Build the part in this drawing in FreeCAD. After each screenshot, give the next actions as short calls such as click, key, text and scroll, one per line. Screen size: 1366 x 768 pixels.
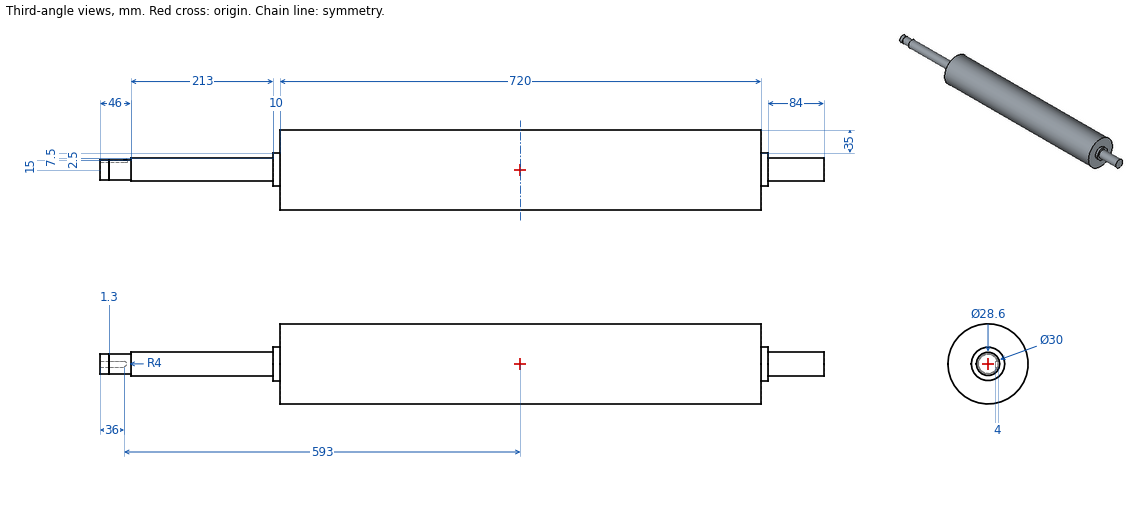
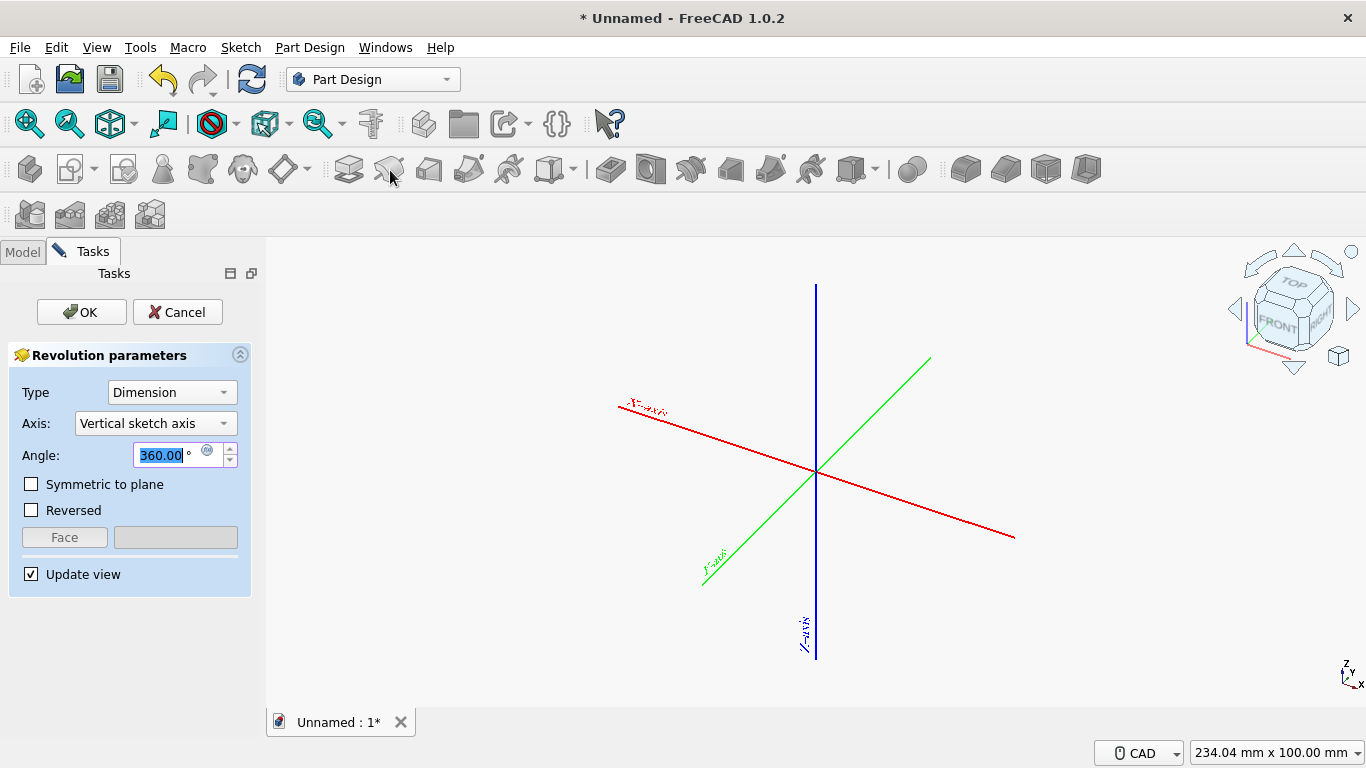
click(156, 424)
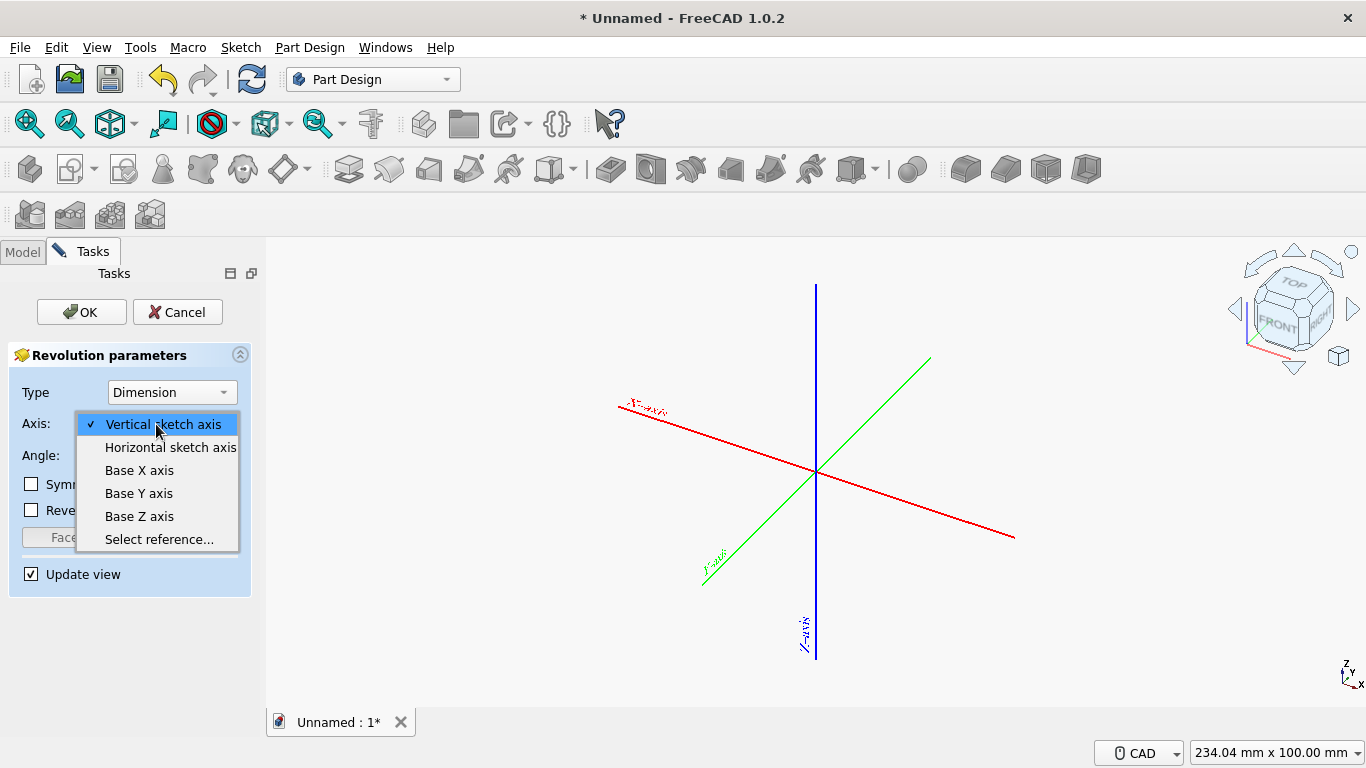
click(156, 448)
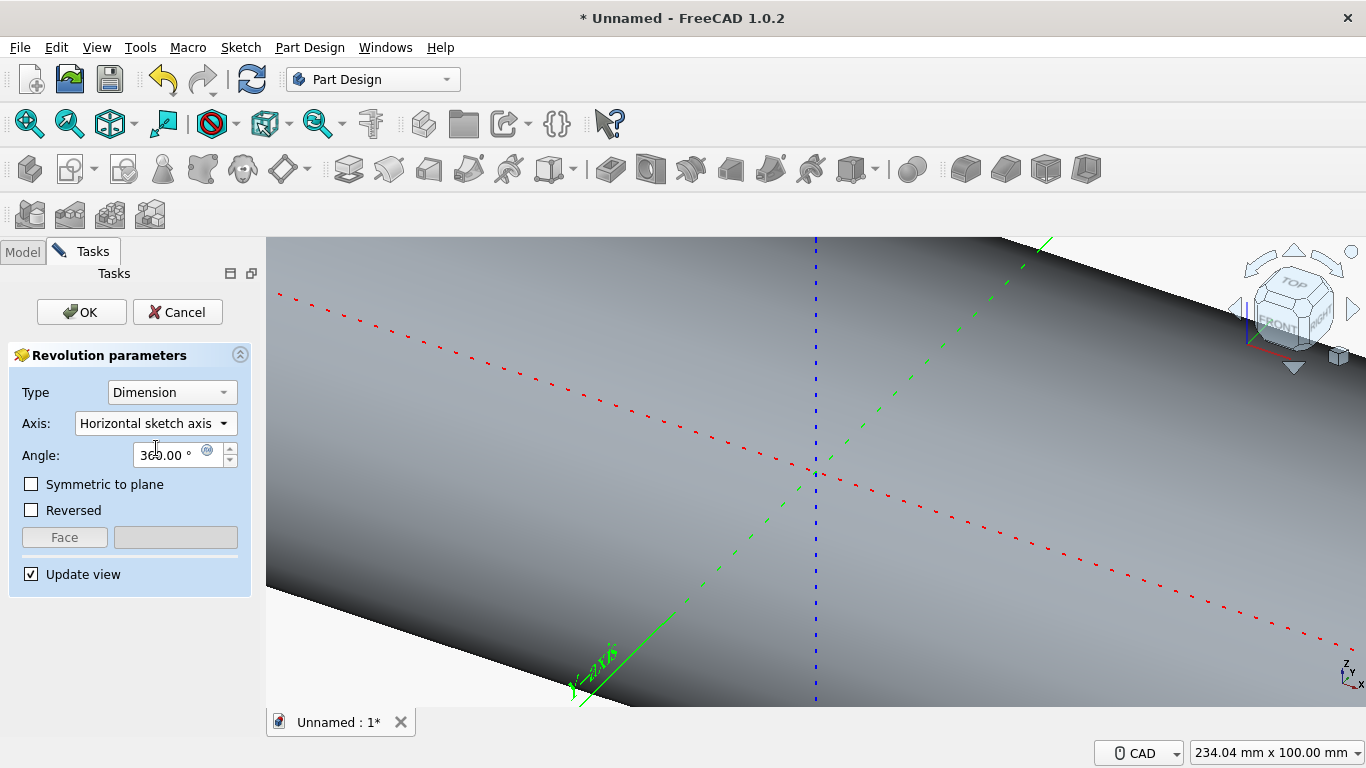
click(82, 312)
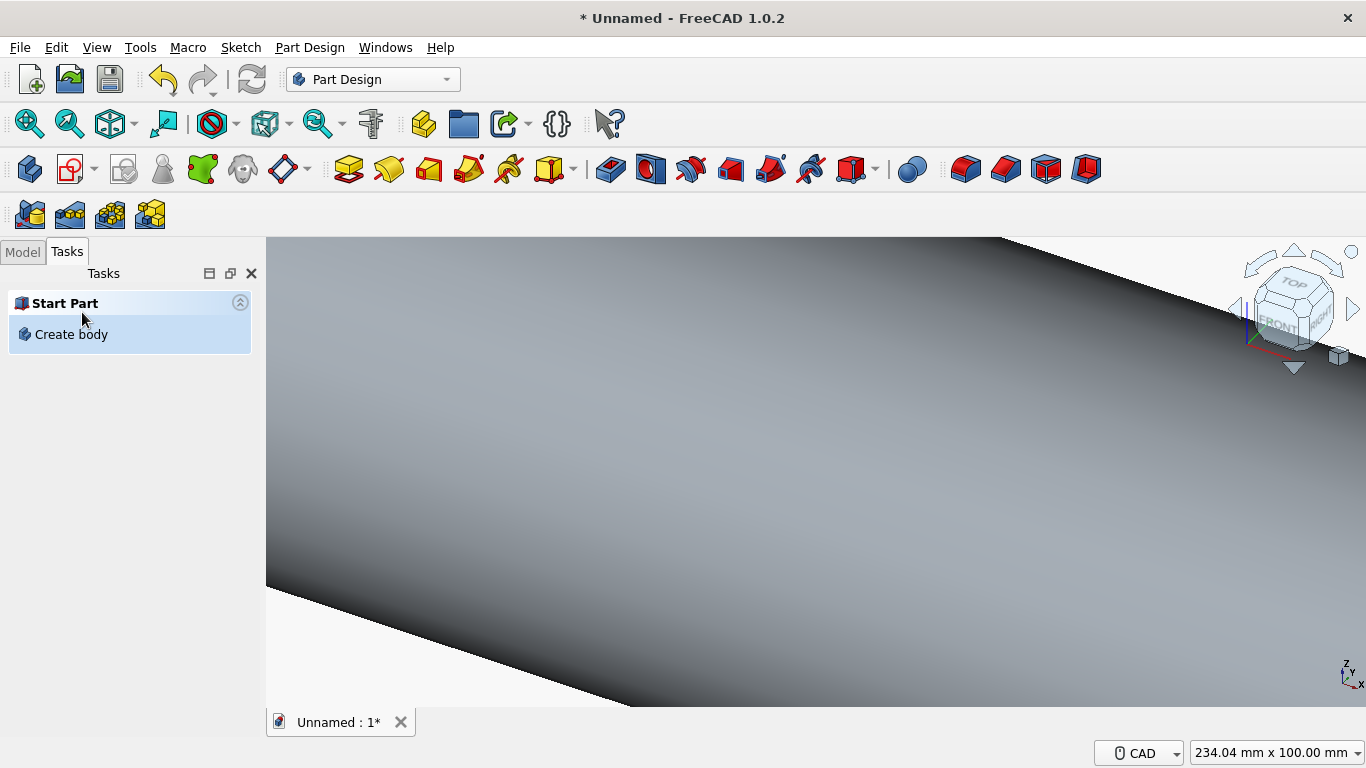
click(30, 124)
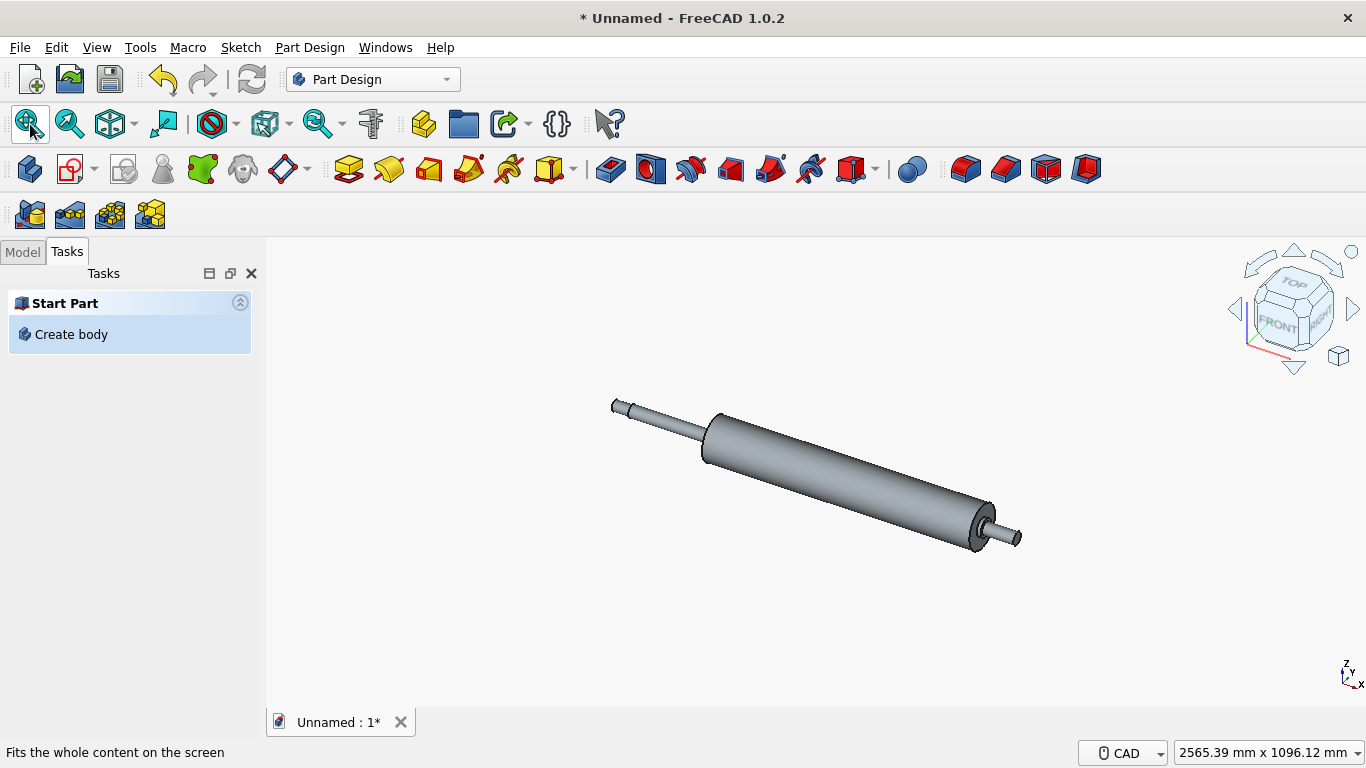
click(23, 251)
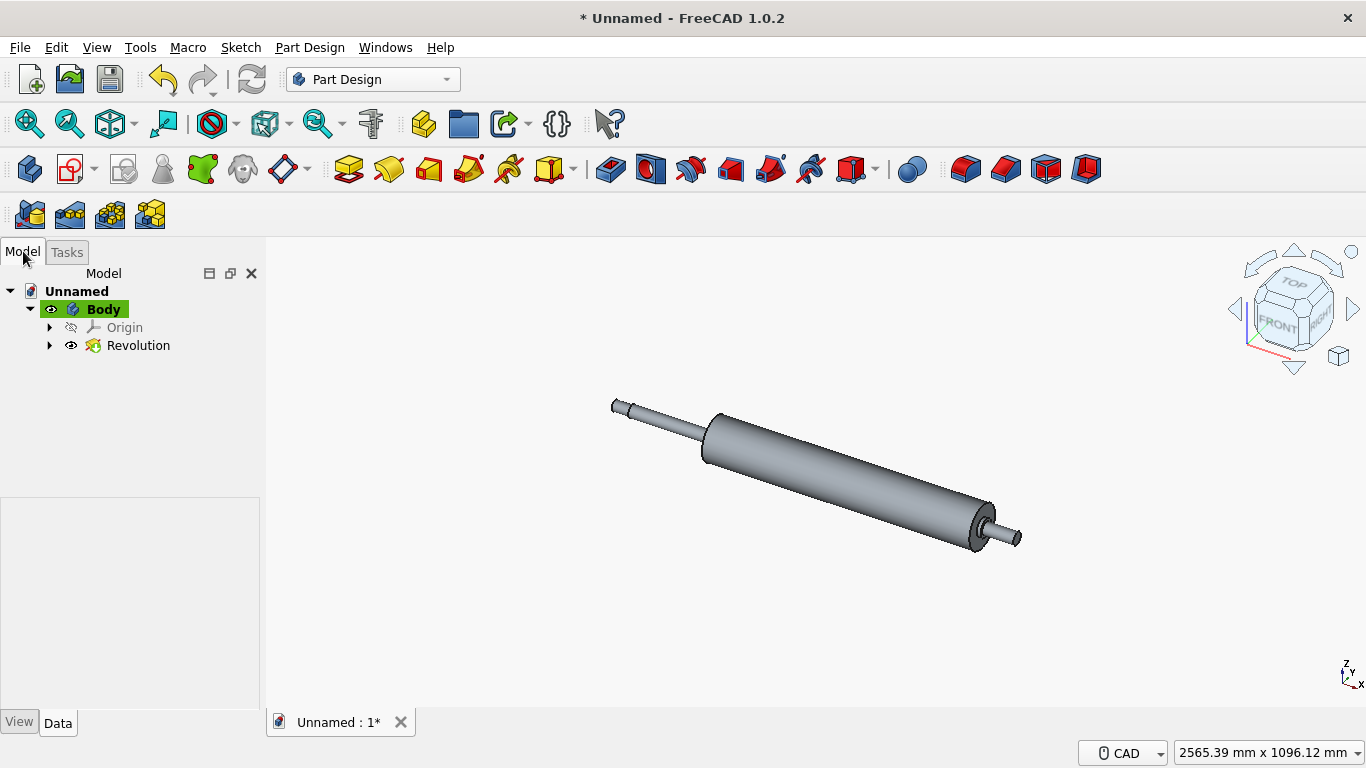
click(50, 327)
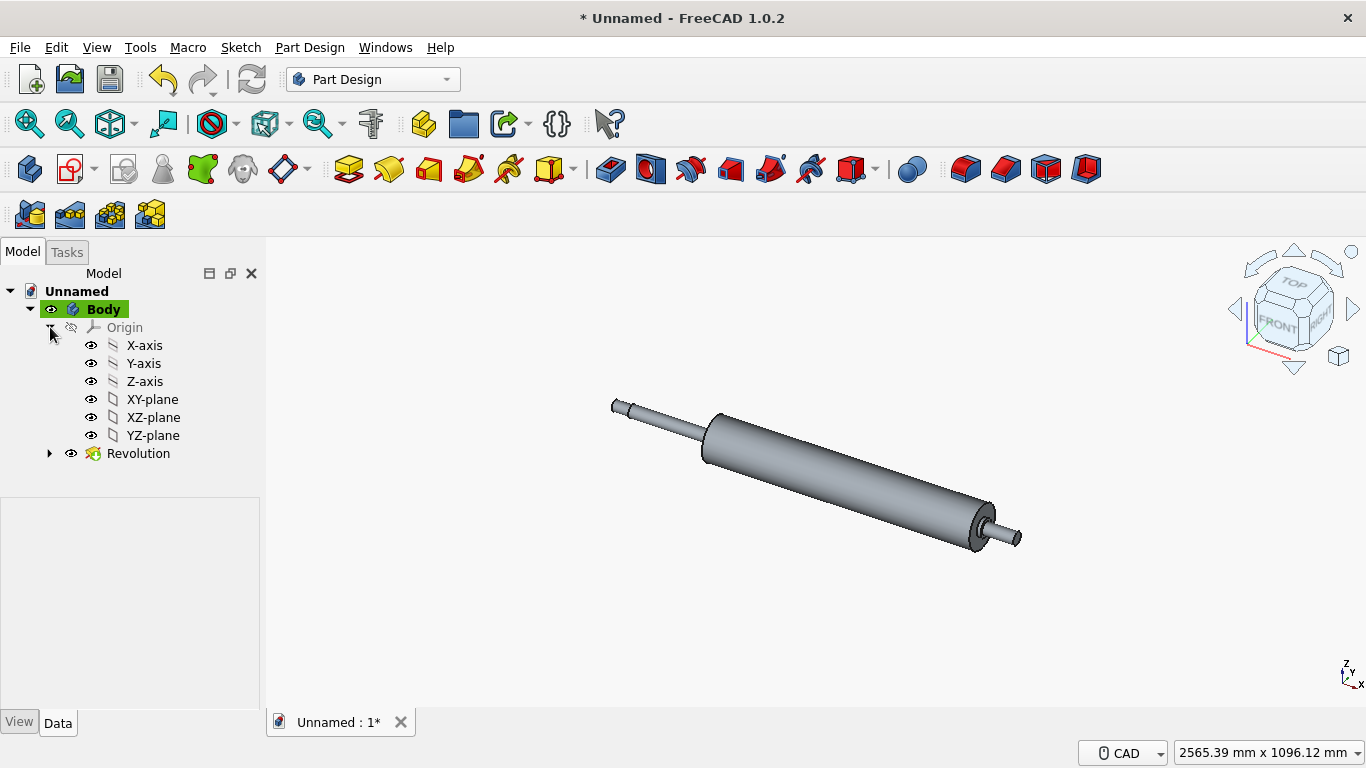
click(136, 417)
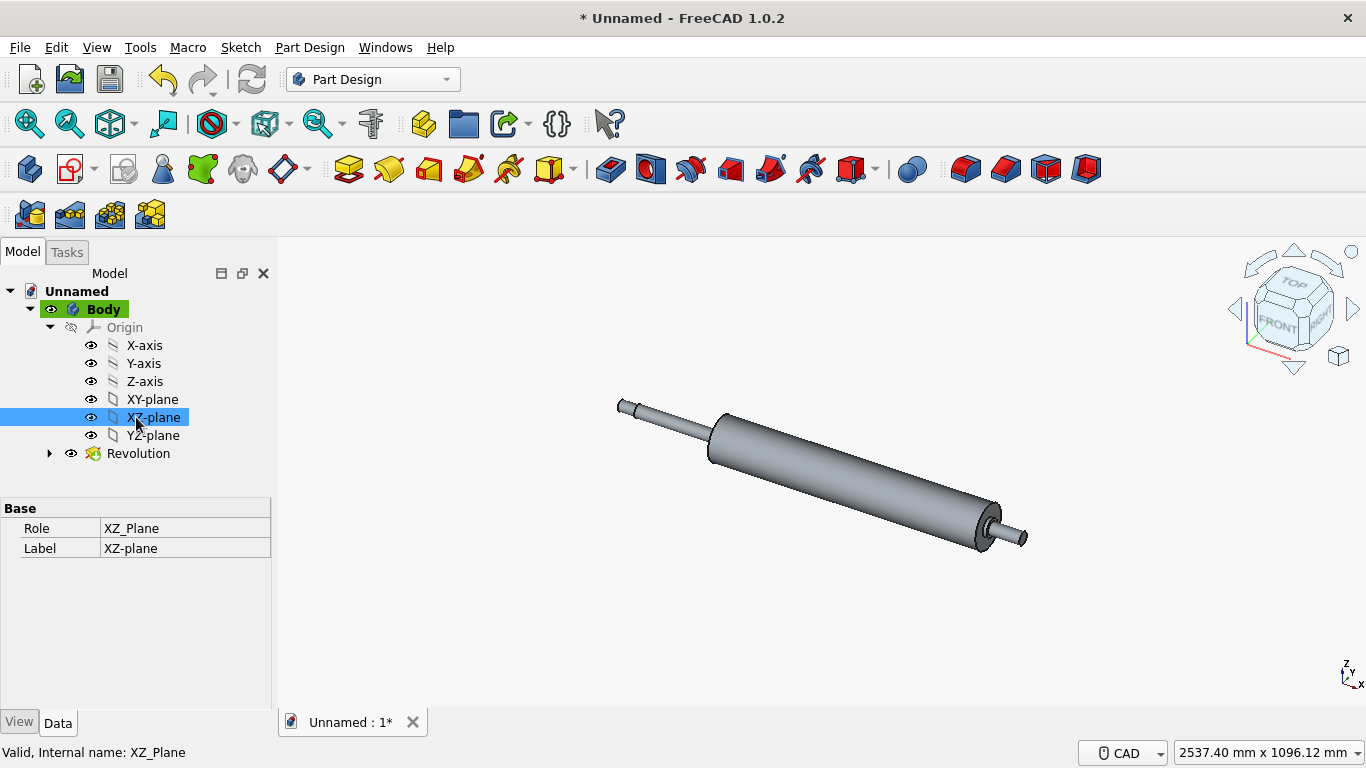
click(284, 170)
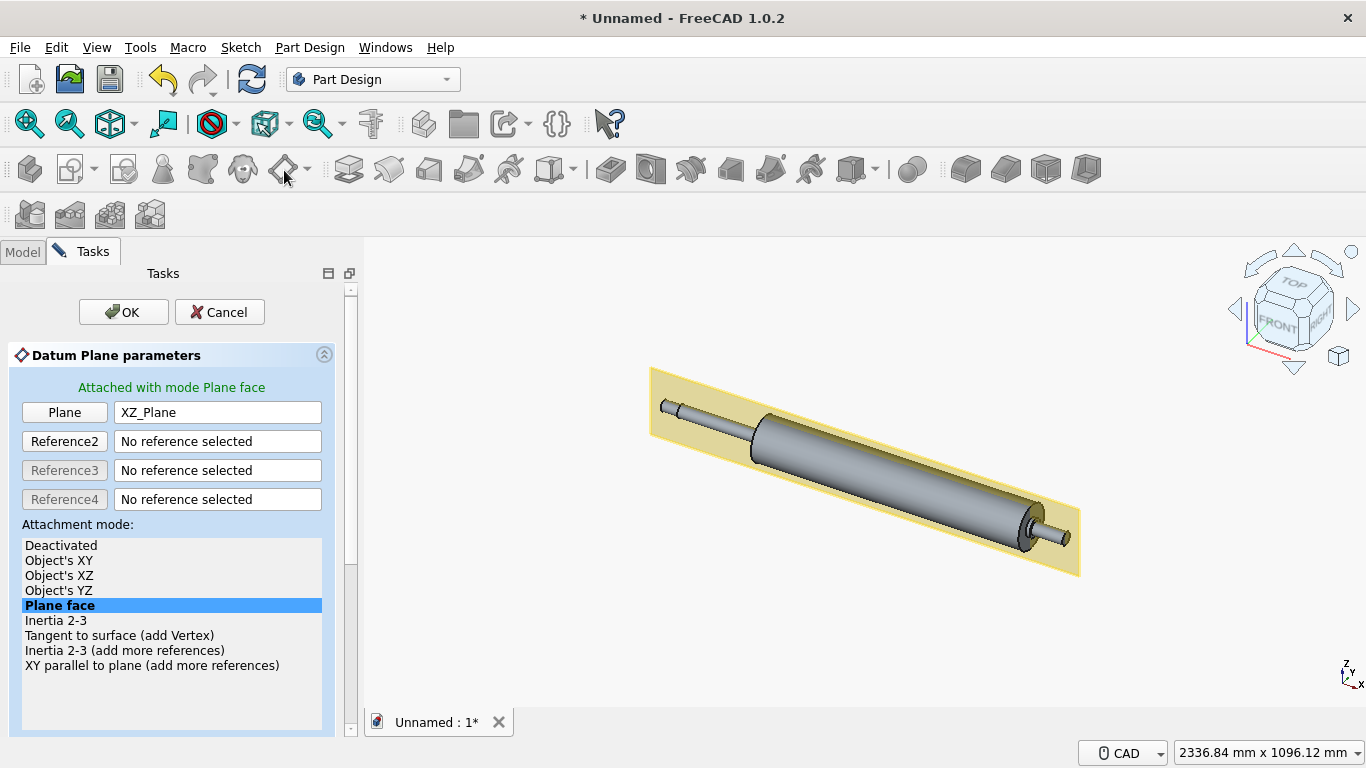
scroll(351, 510, down, 3)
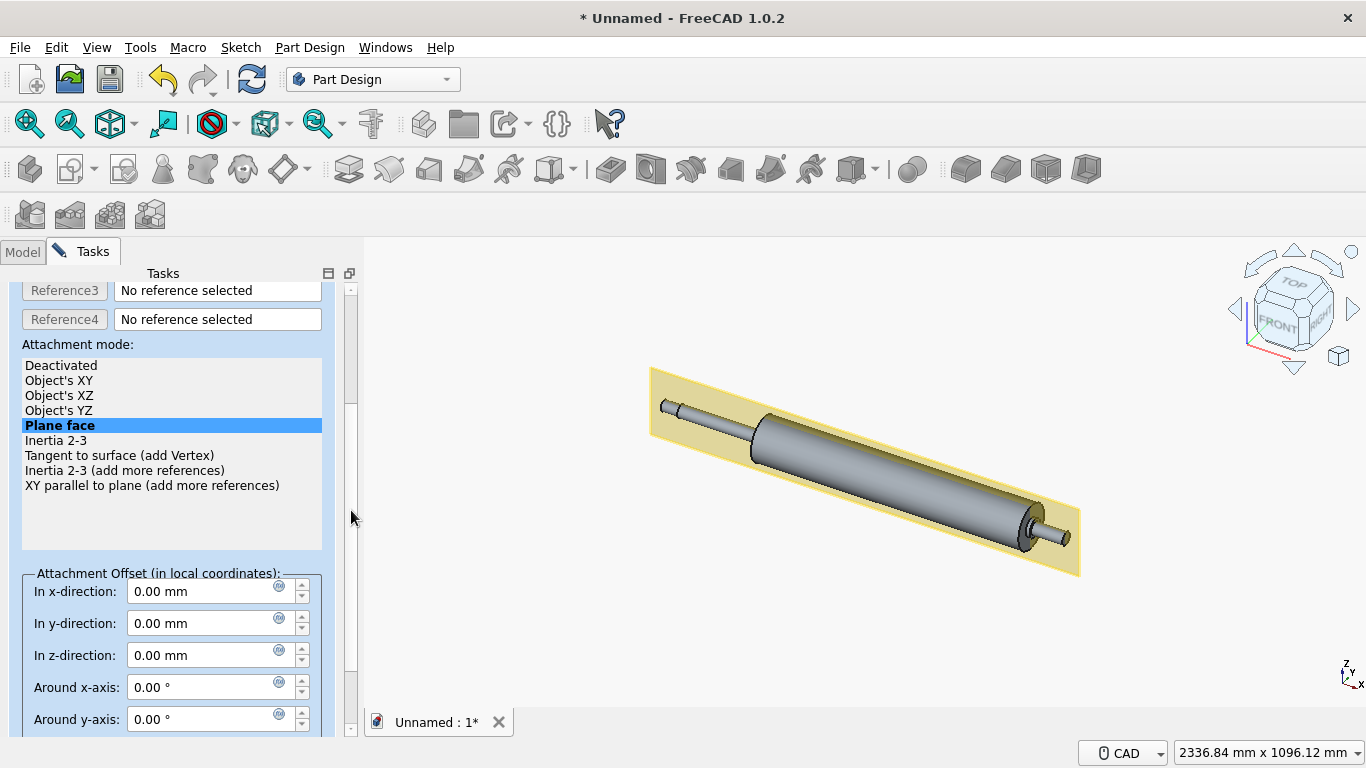
triple_click(210, 655)